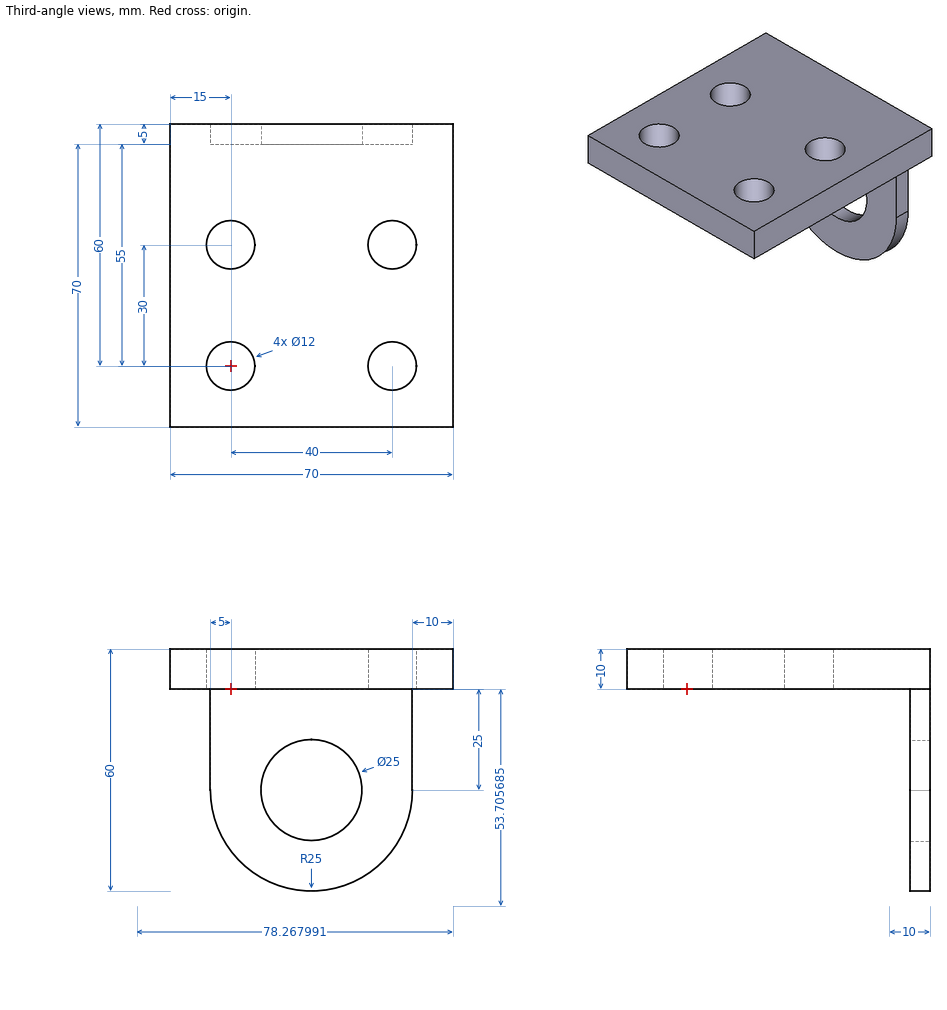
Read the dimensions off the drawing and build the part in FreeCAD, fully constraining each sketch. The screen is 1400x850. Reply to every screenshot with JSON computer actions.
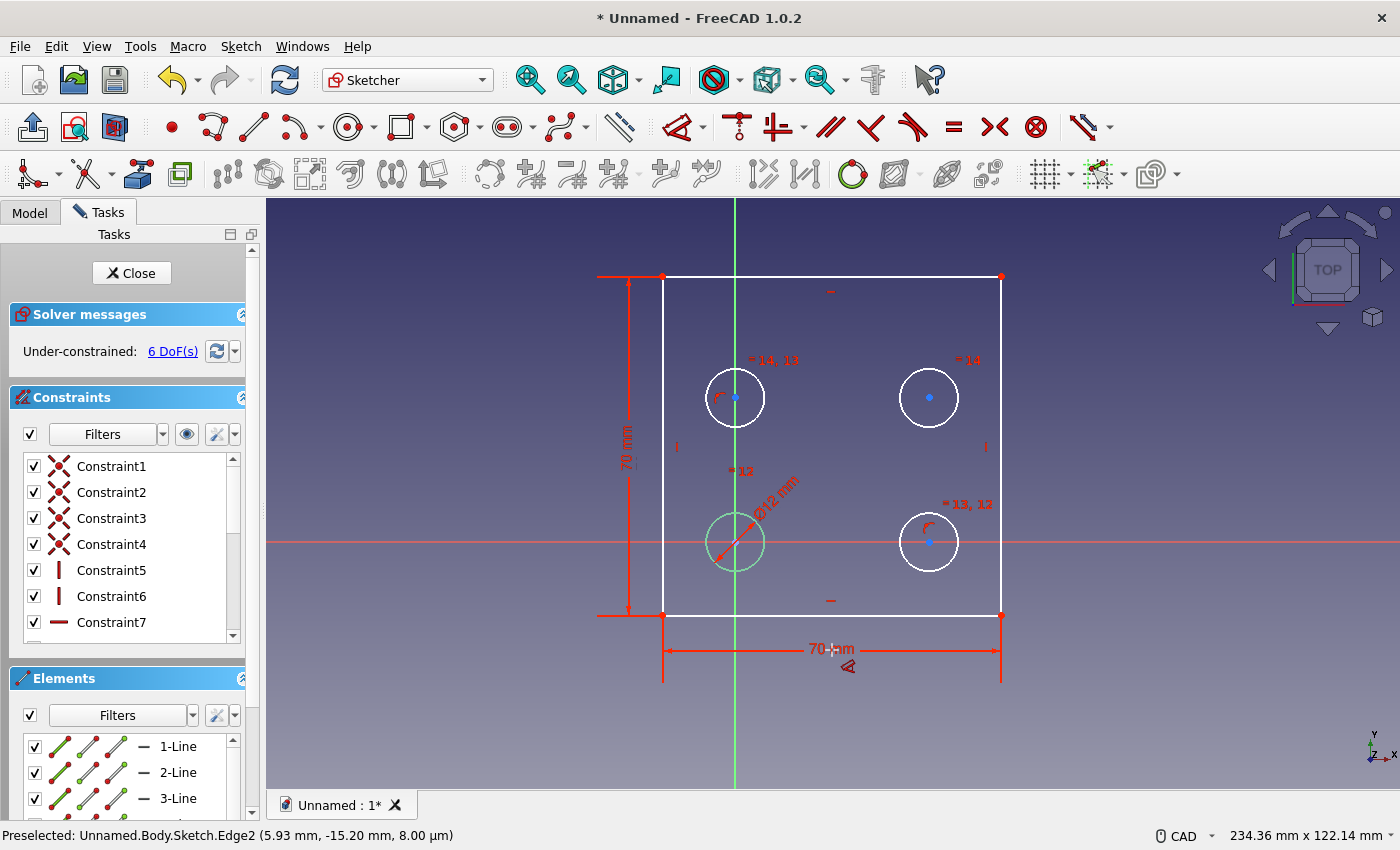
{"action": "left_click", "coordinate": [929, 542]}
{"action": "left_click", "coordinate": [832, 576]}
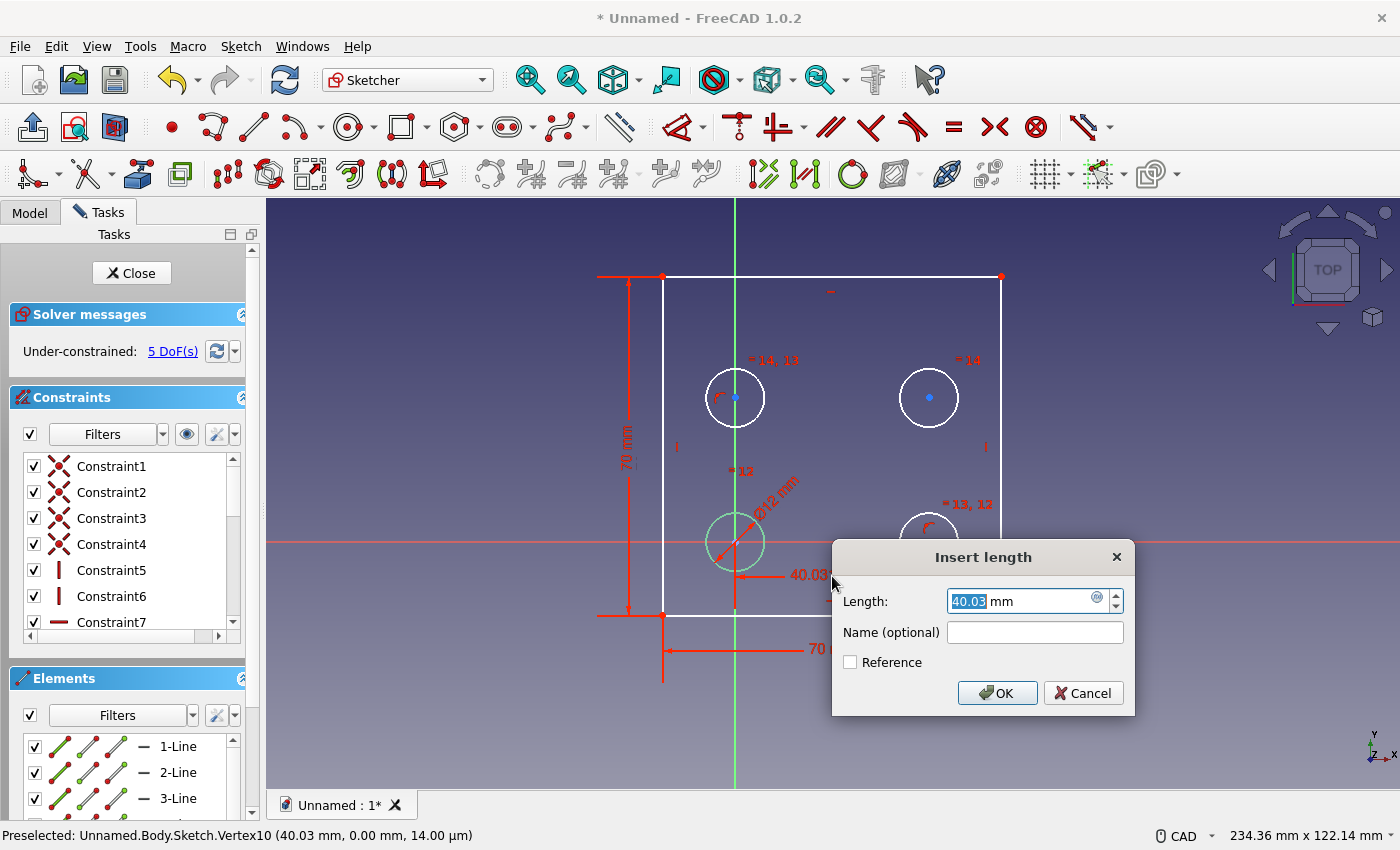
{"action": "type", "text": "40"}
{"action": "key", "text": "Return"}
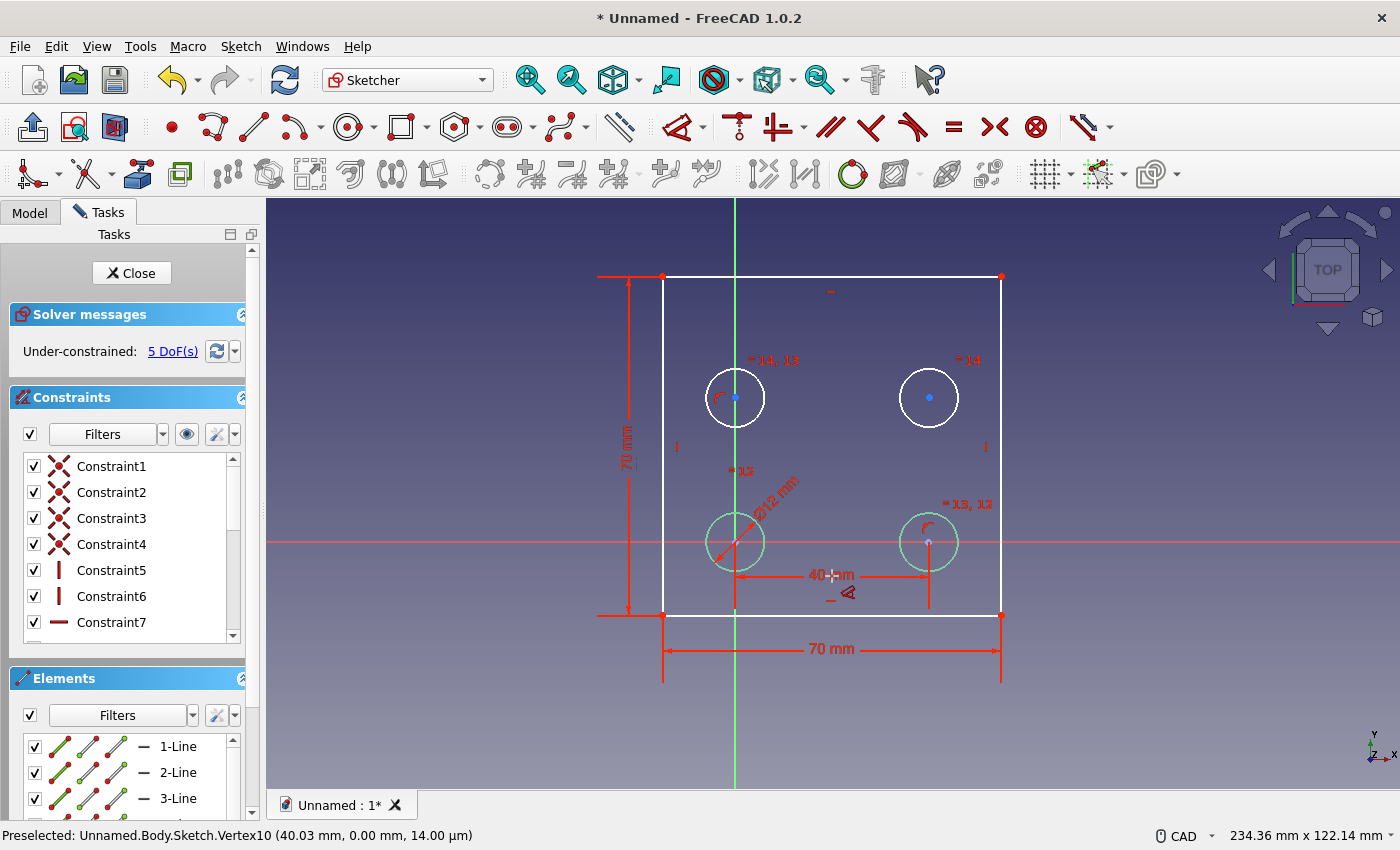
{"action": "left_click", "coordinate": [735, 398]}
{"action": "left_click", "coordinate": [701, 470]}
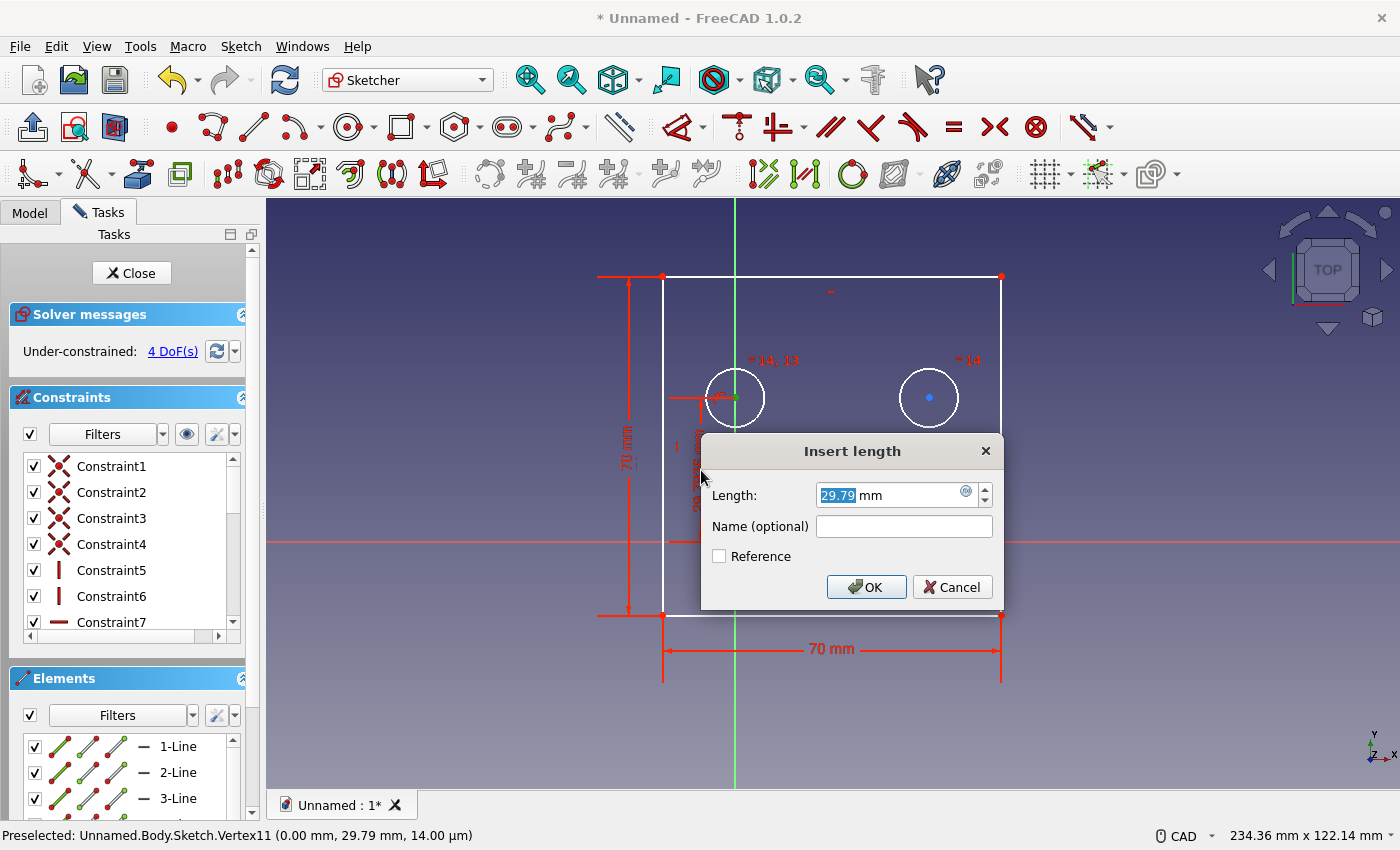
{"action": "type", "text": "30"}
{"action": "key", "text": "Return"}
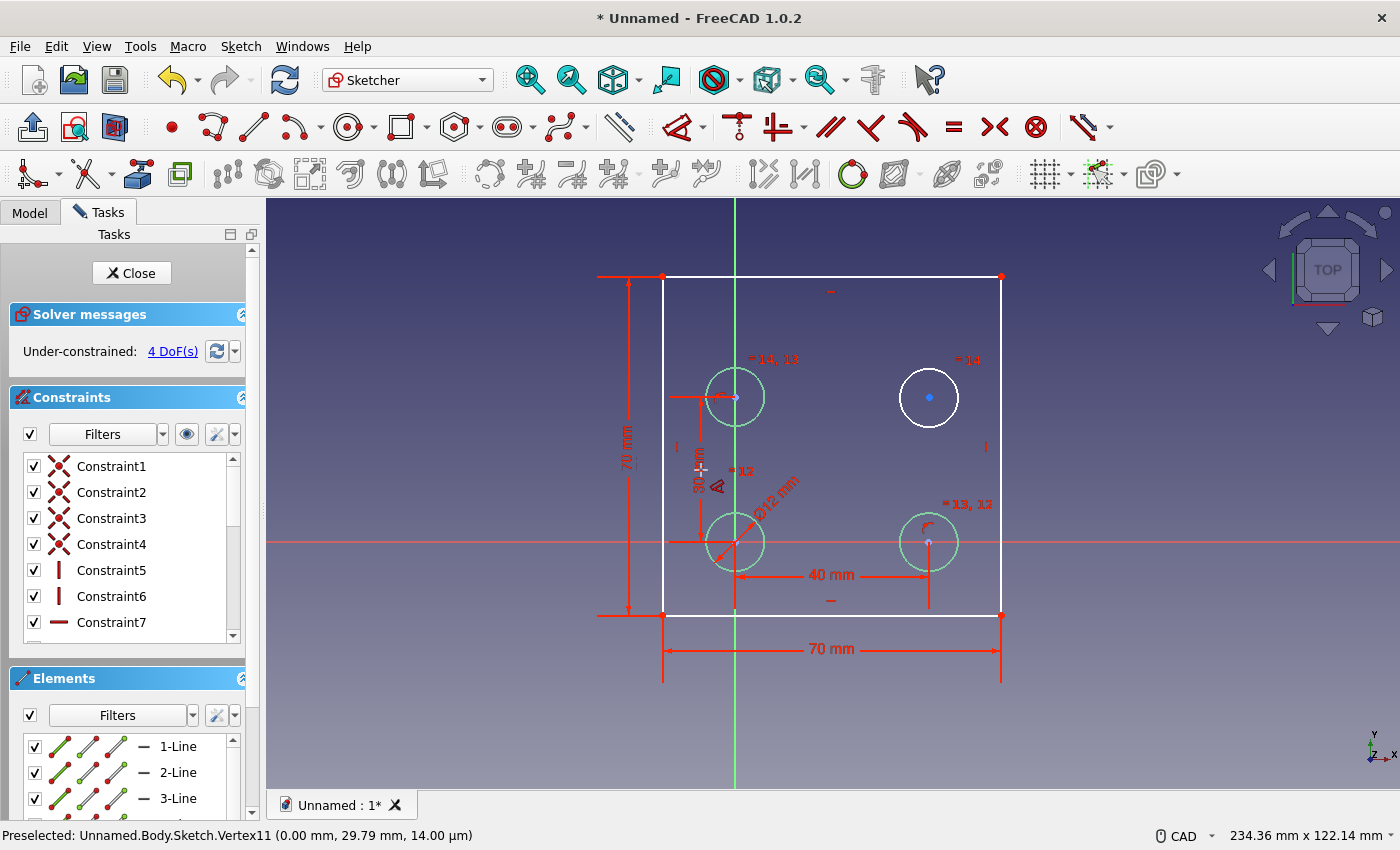
{"action": "left_click", "coordinate": [929, 398]}
{"action": "left_click", "coordinate": [832, 364]}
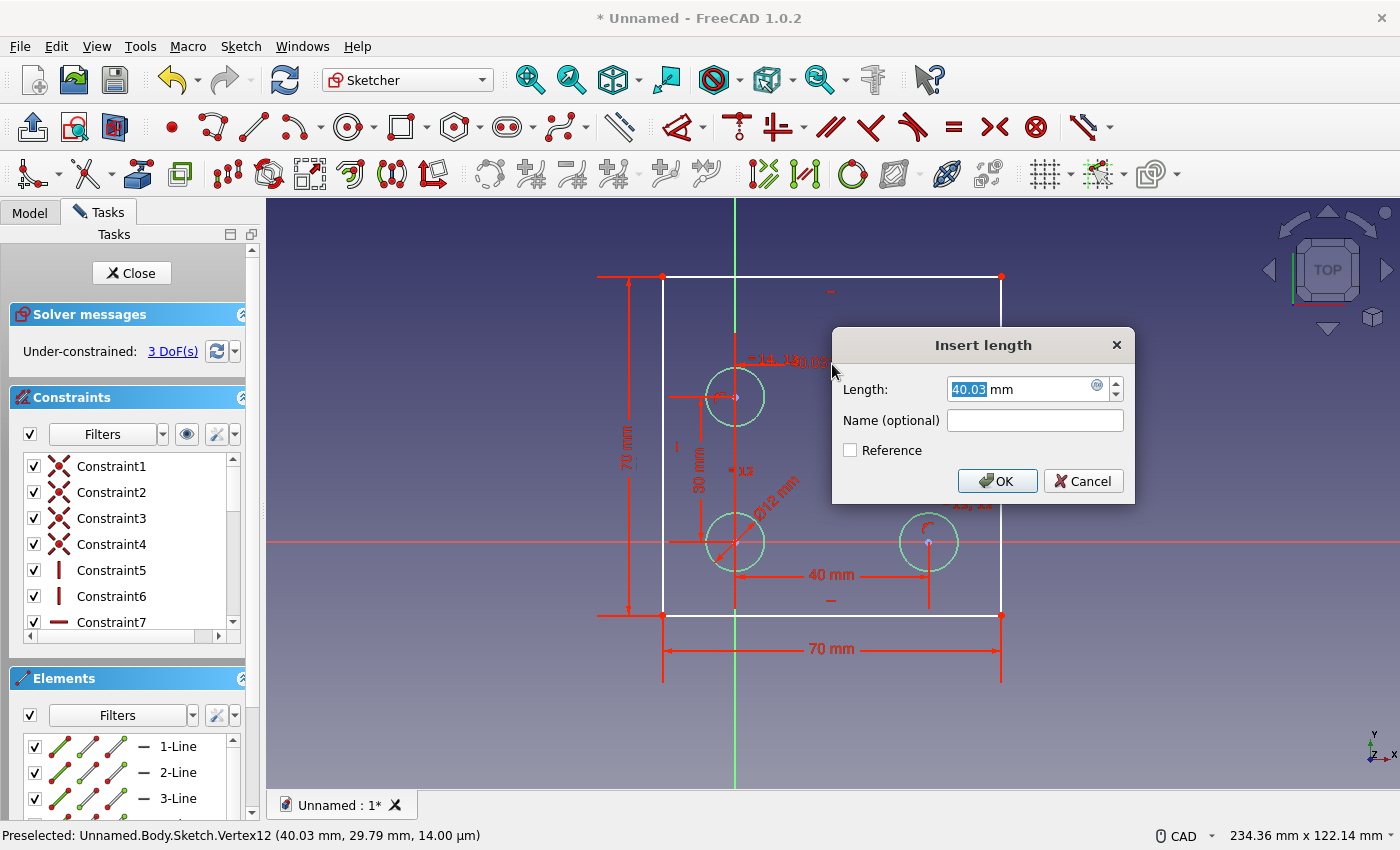
{"action": "type", "text": "40"}
{"action": "key", "text": "Return"}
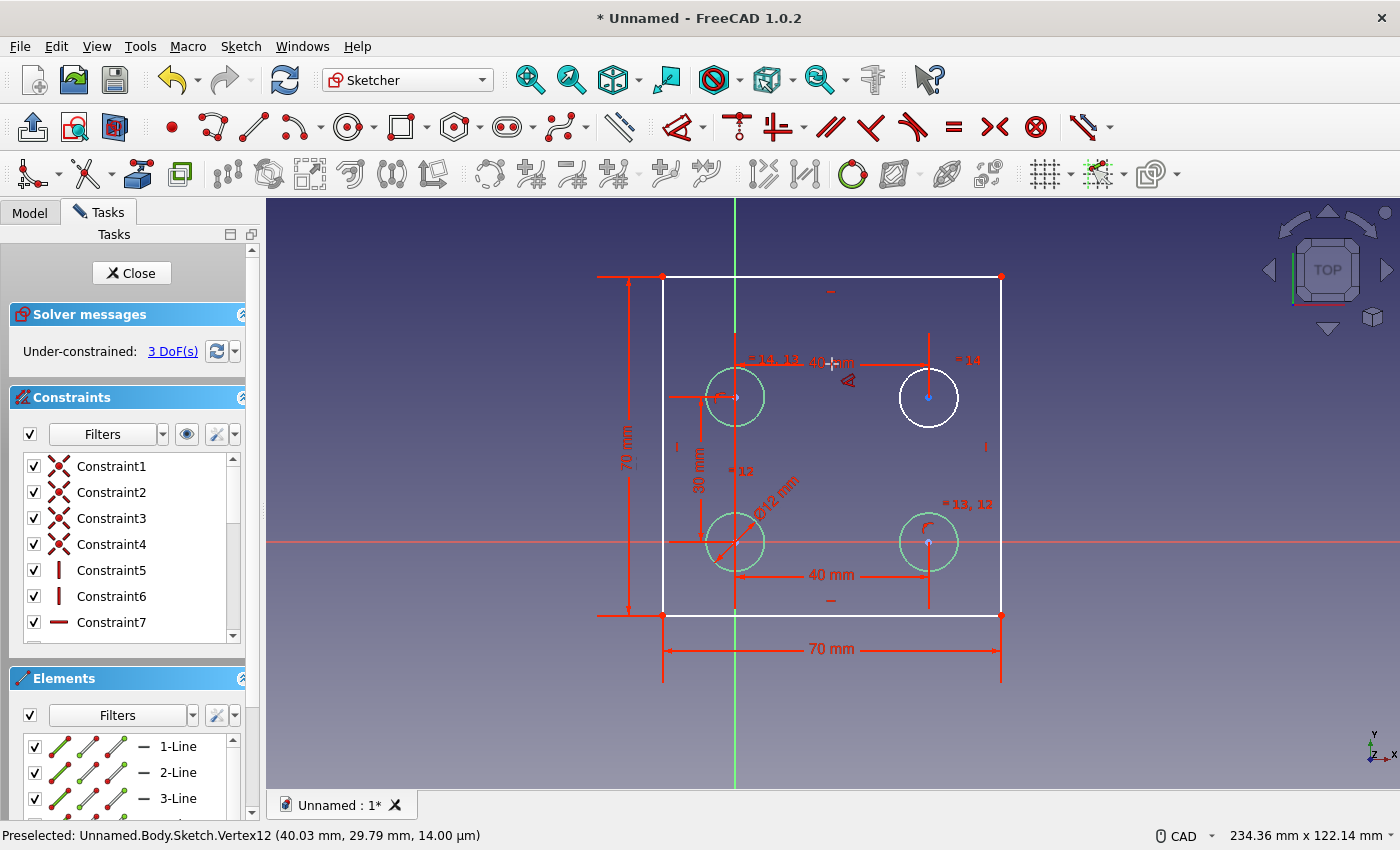
{"action": "left_click", "coordinate": [929, 398]}
{"action": "left_click", "coordinate": [963, 470]}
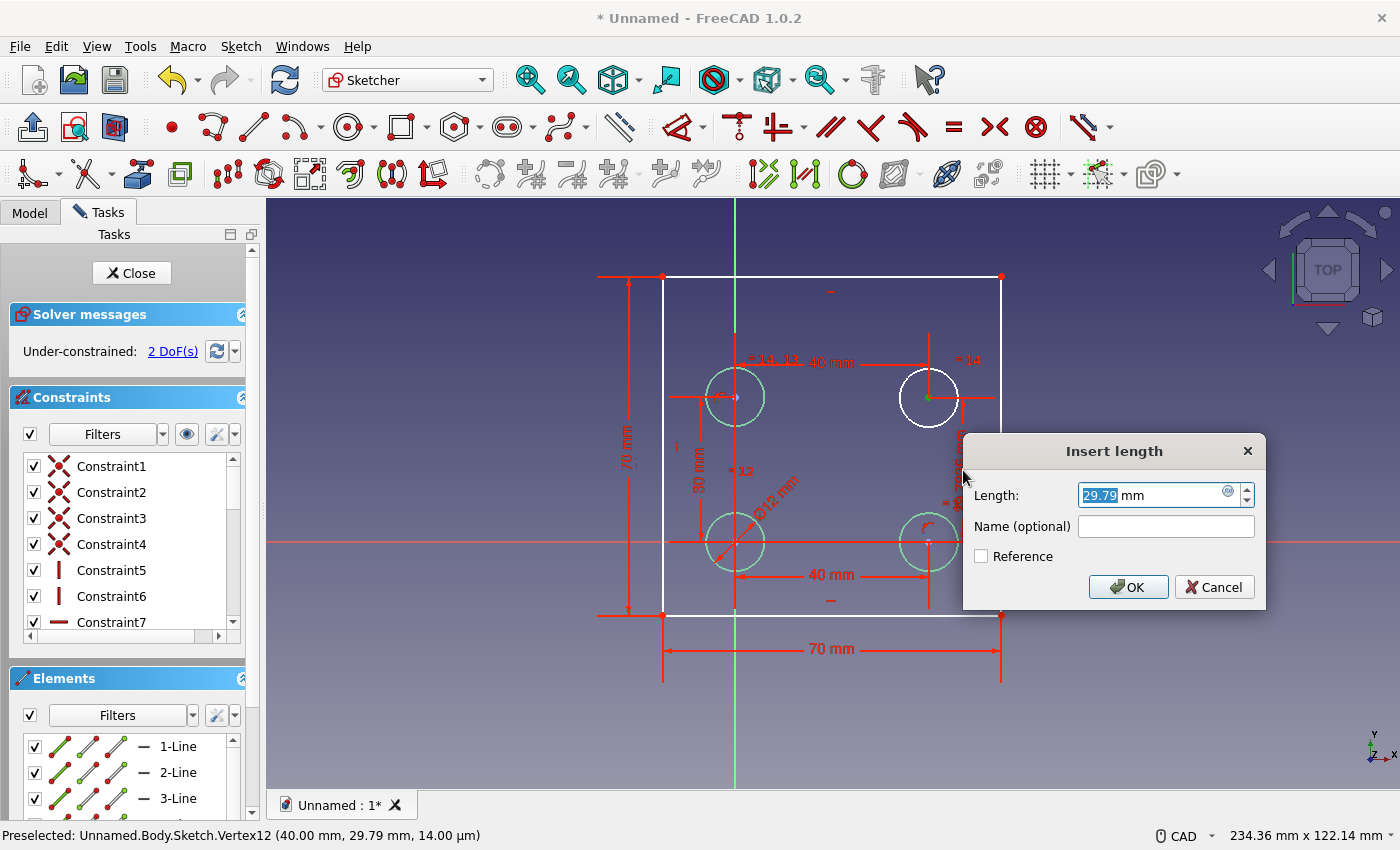
{"action": "type", "text": "30"}
{"action": "key", "text": "Return"}